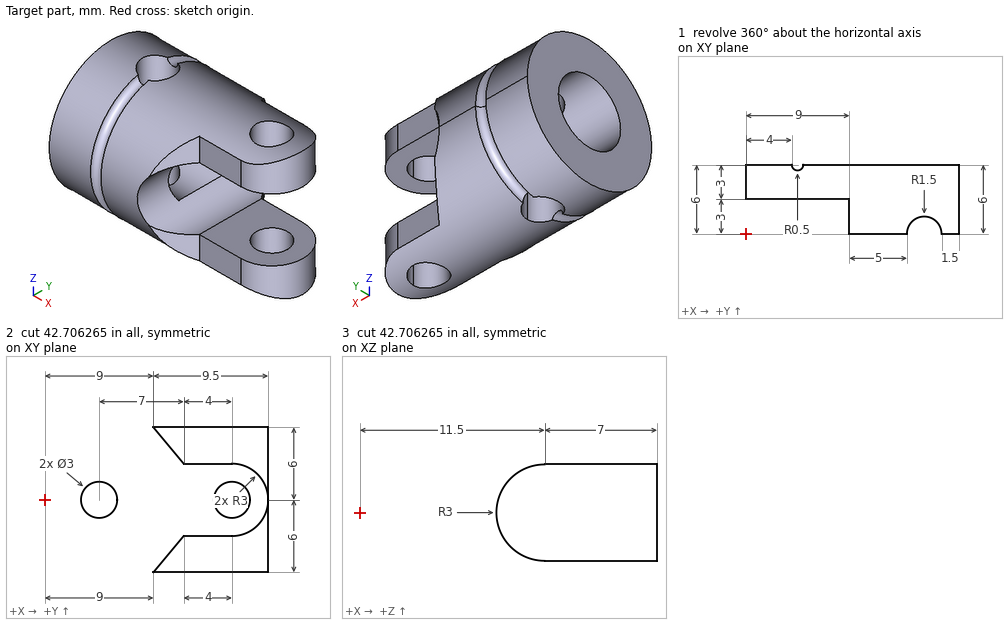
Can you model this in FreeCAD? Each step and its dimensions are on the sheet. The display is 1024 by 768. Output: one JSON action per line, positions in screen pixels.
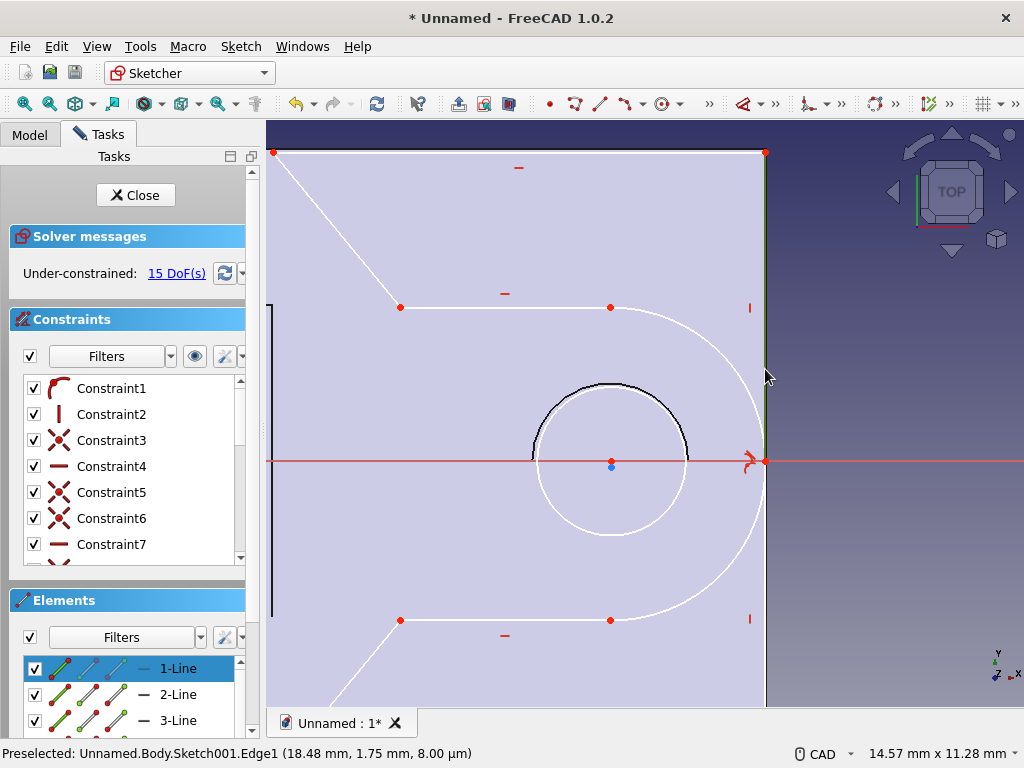
{"action": "left_click", "coordinate": [682, 603]}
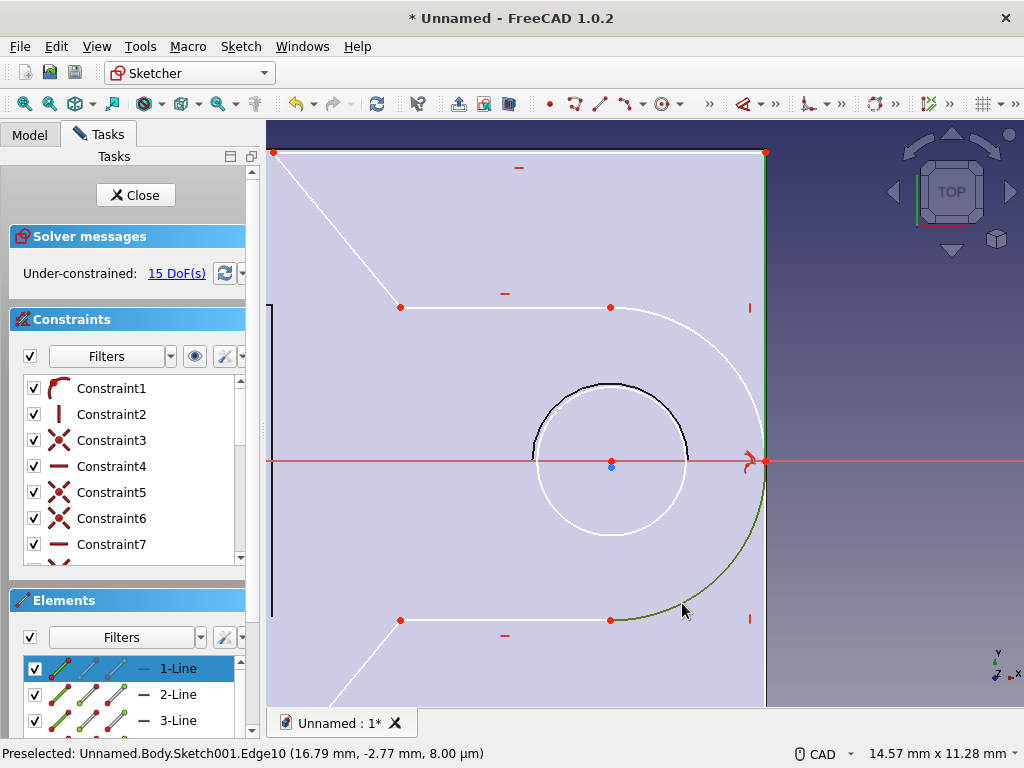
{"action": "key", "text": "t"}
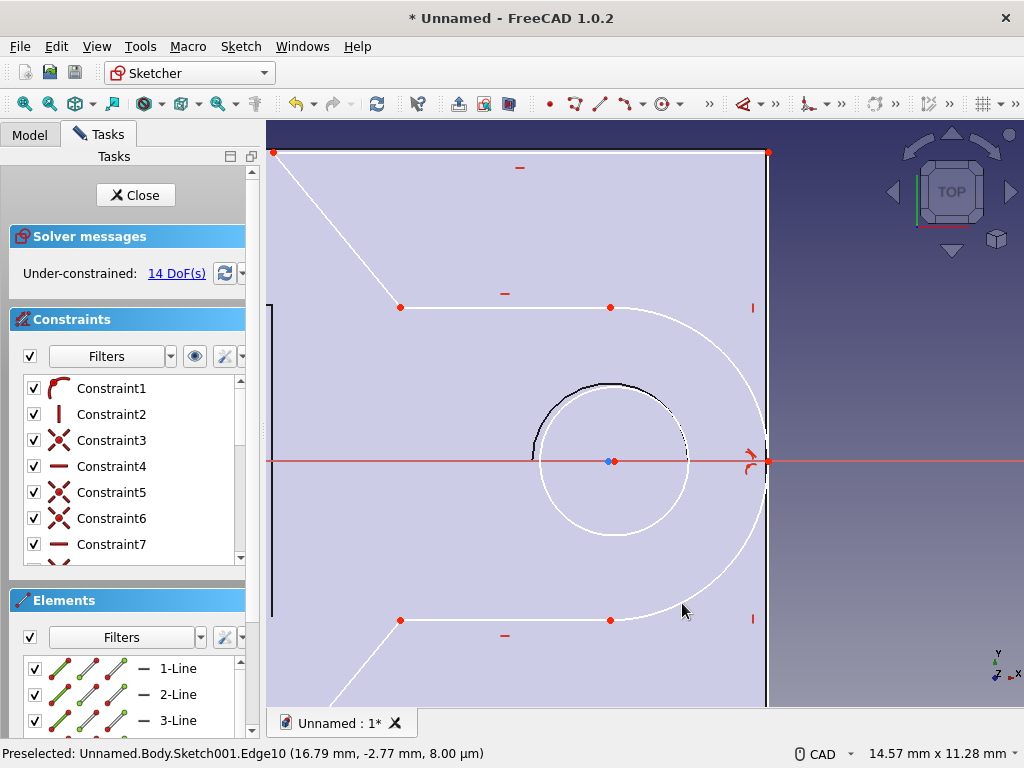
{"action": "left_click", "coordinate": [464, 308]}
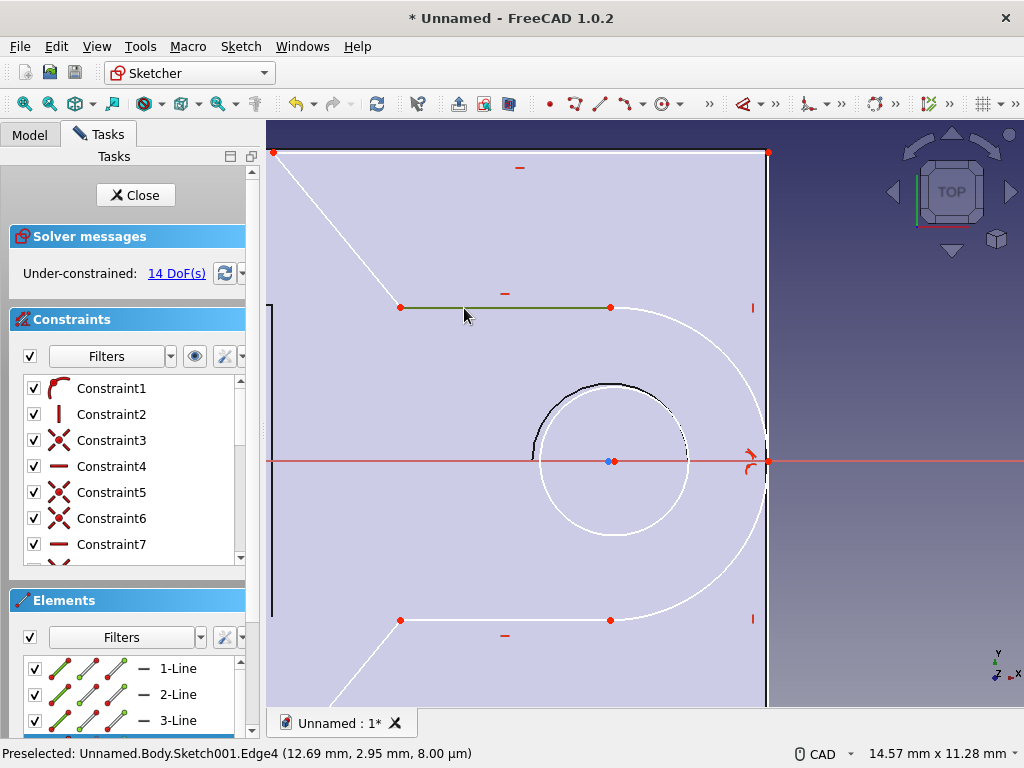
{"action": "left_click", "coordinate": [751, 390]}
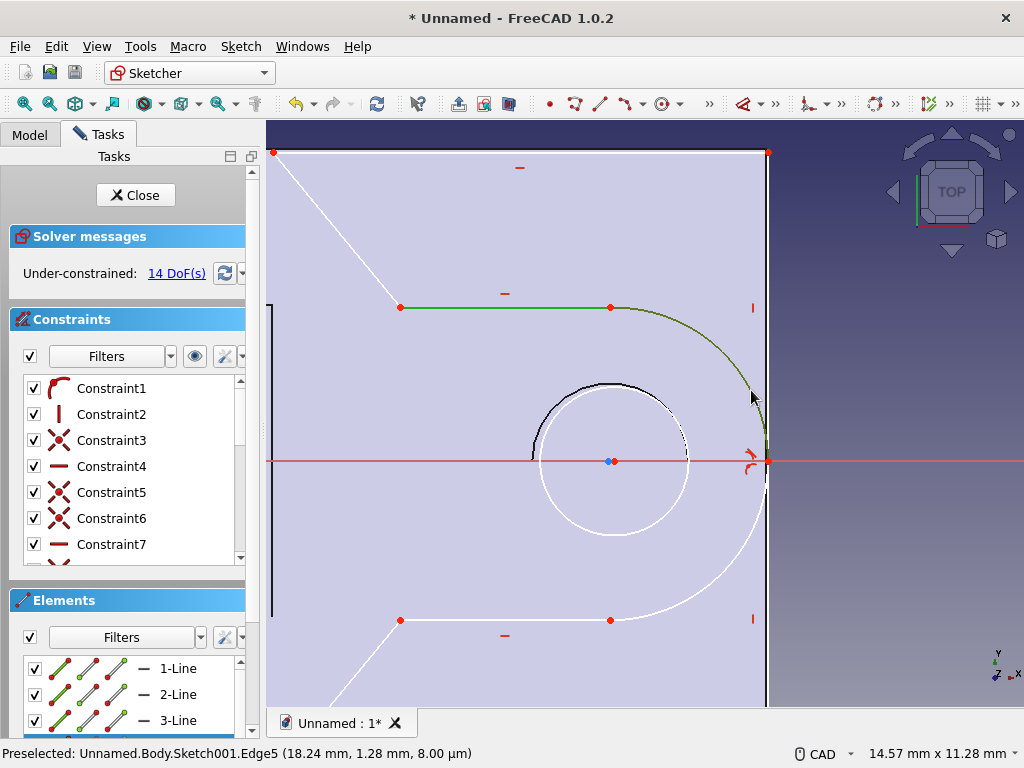
{"action": "key", "text": "t"}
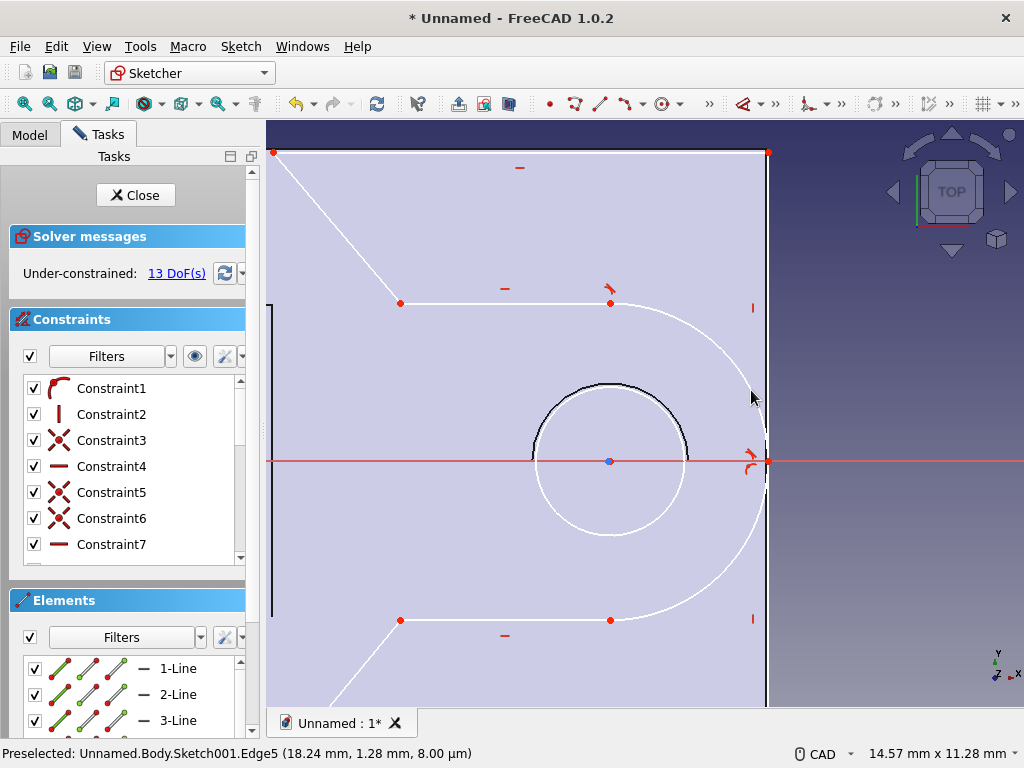
{"action": "left_click", "coordinate": [547, 620]}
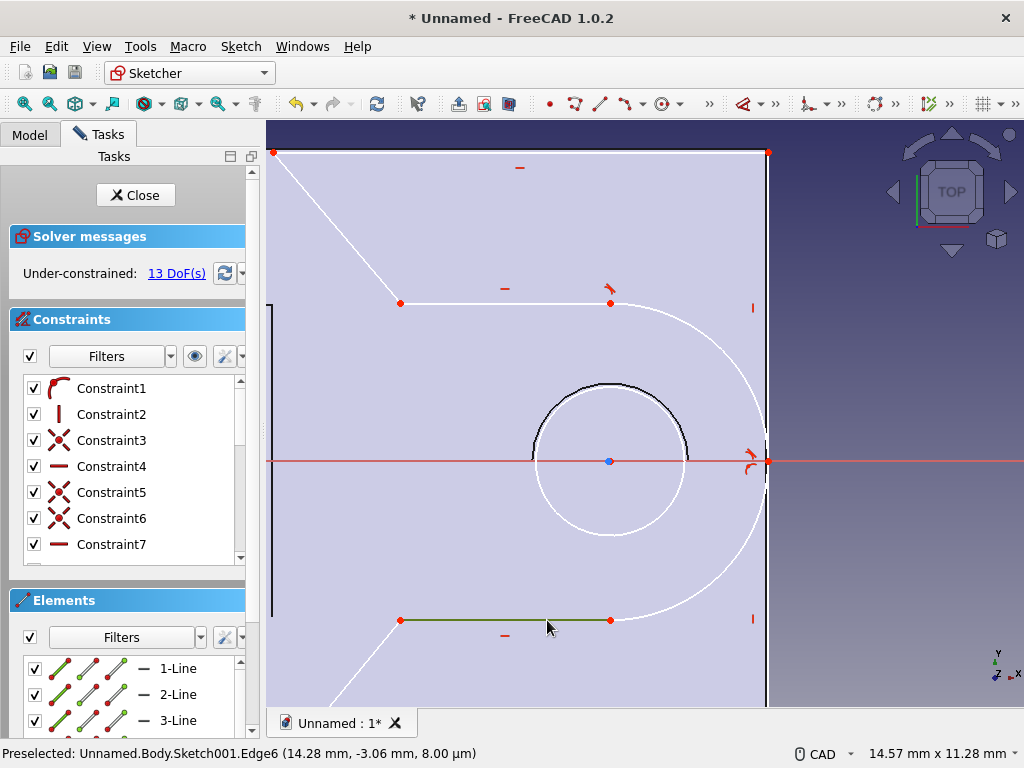
{"action": "left_click", "coordinate": [682, 603]}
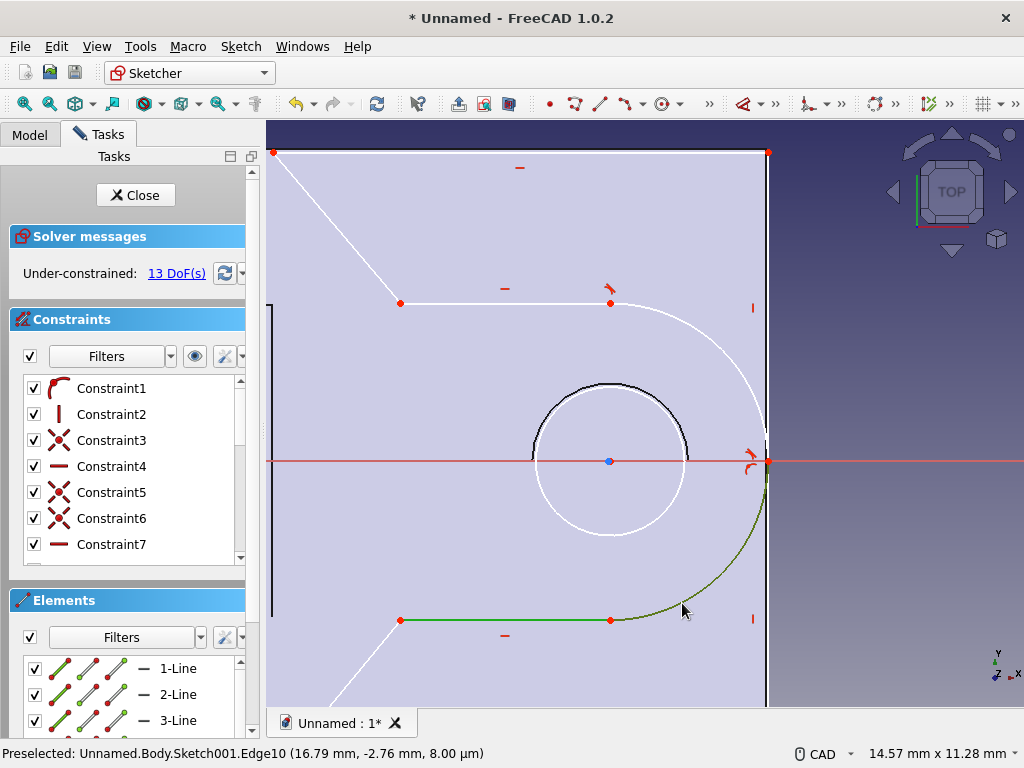
{"action": "key", "text": "t"}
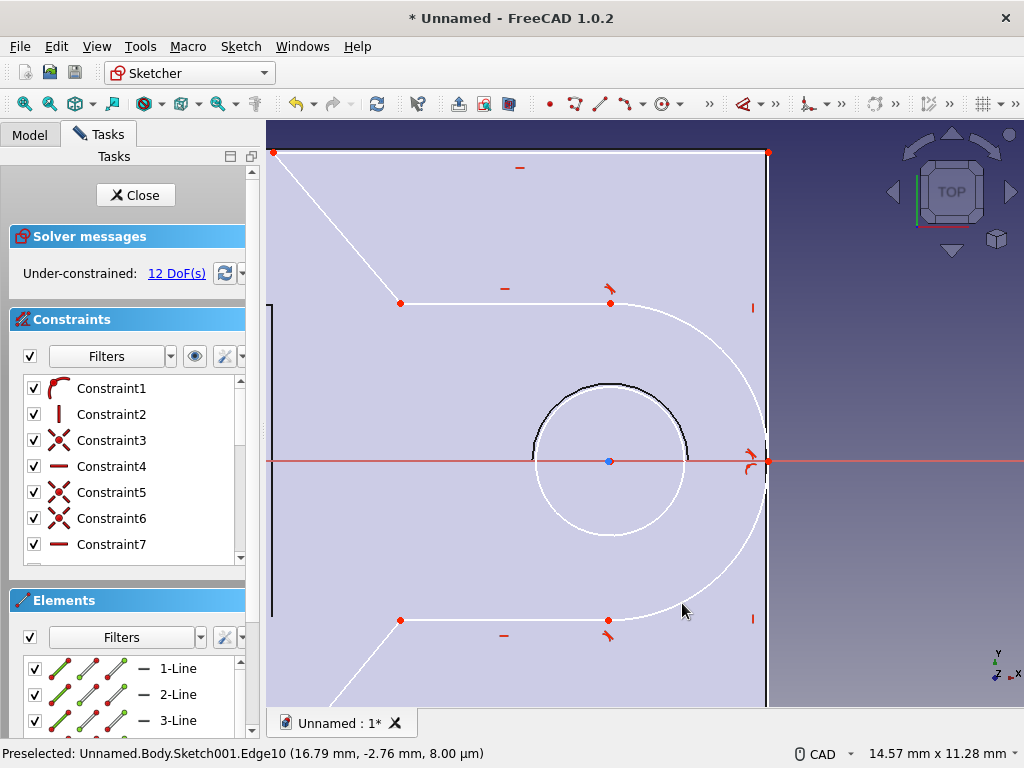
{"action": "left_click", "coordinate": [751, 390]}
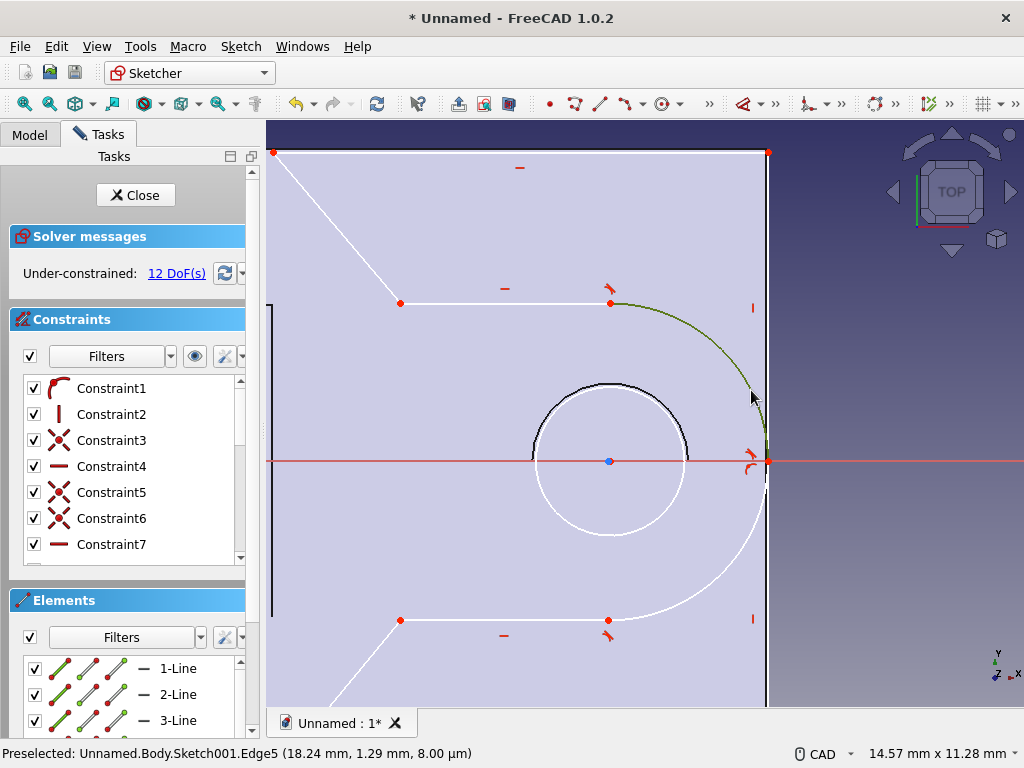
{"action": "left_click", "coordinate": [681, 603]}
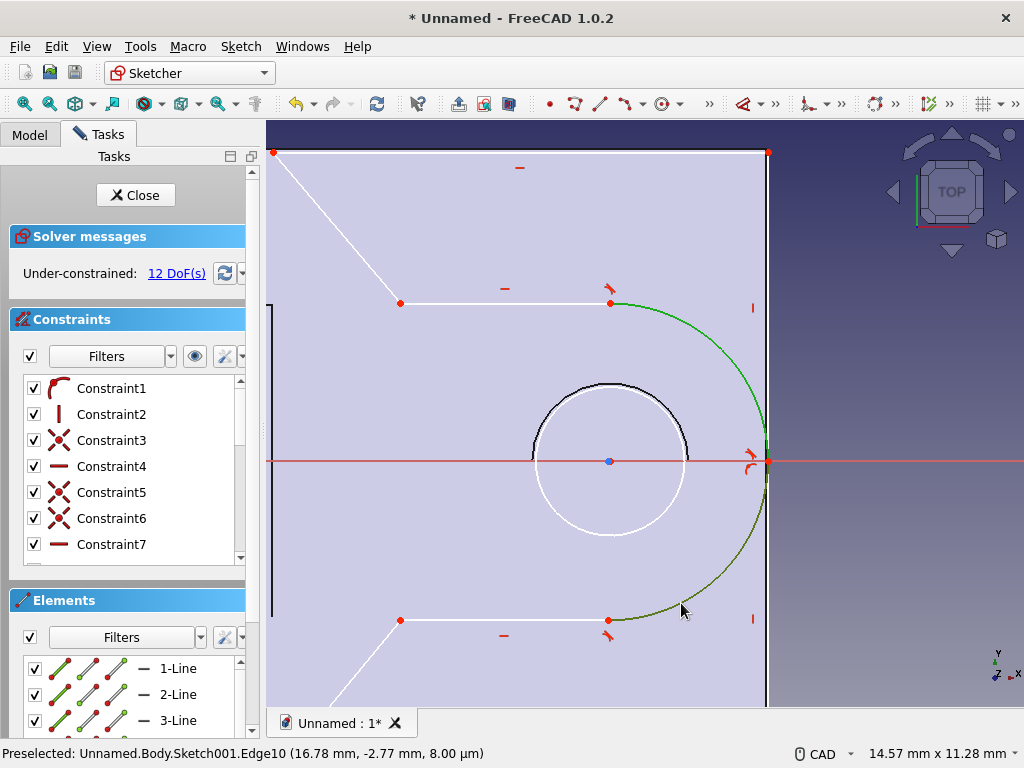
{"action": "key", "text": "e"}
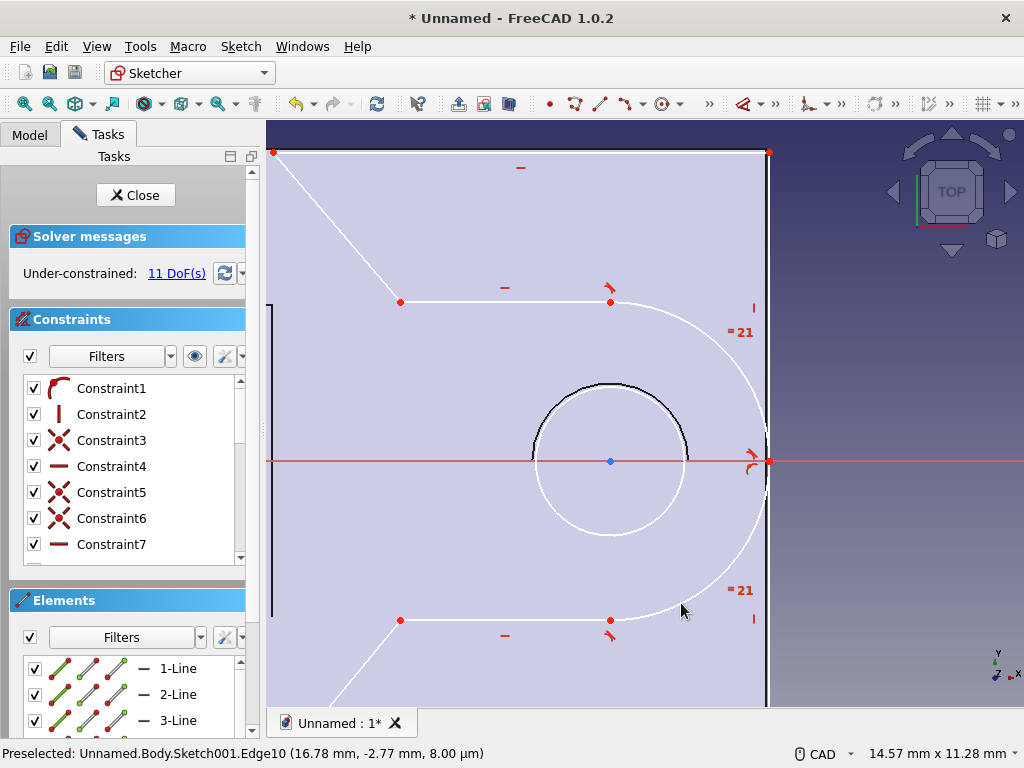
{"action": "left_click", "coordinate": [663, 409]}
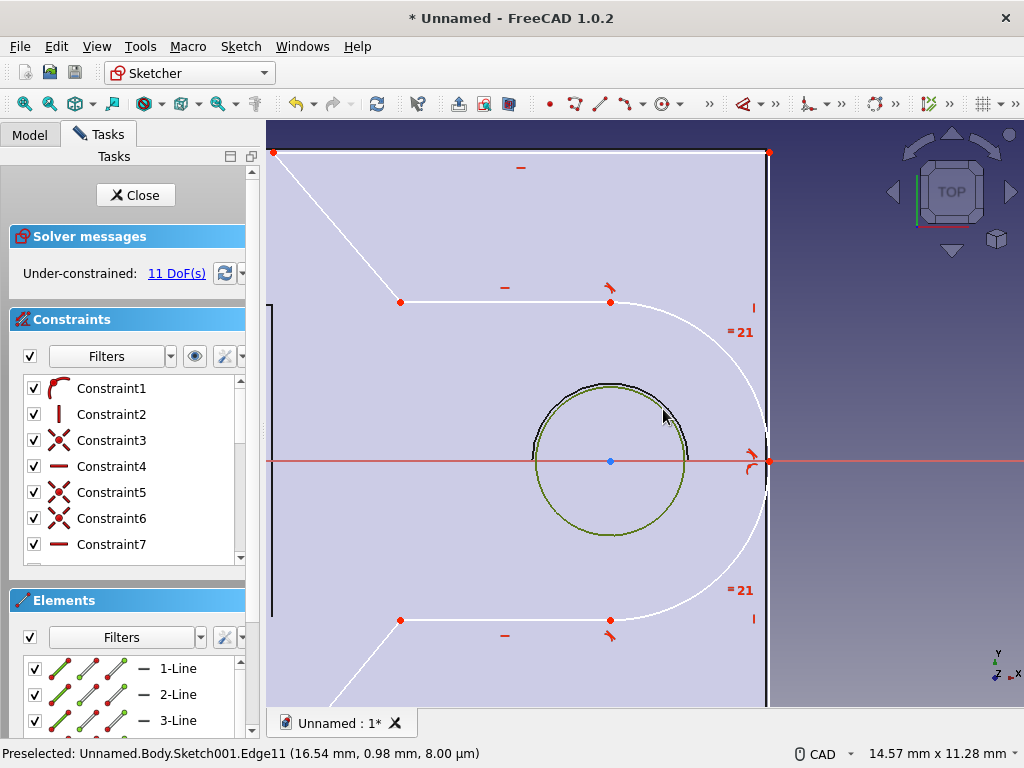
{"action": "scroll", "coordinate": [814, 374], "scroll_direction": "down", "scroll_amount": 4}